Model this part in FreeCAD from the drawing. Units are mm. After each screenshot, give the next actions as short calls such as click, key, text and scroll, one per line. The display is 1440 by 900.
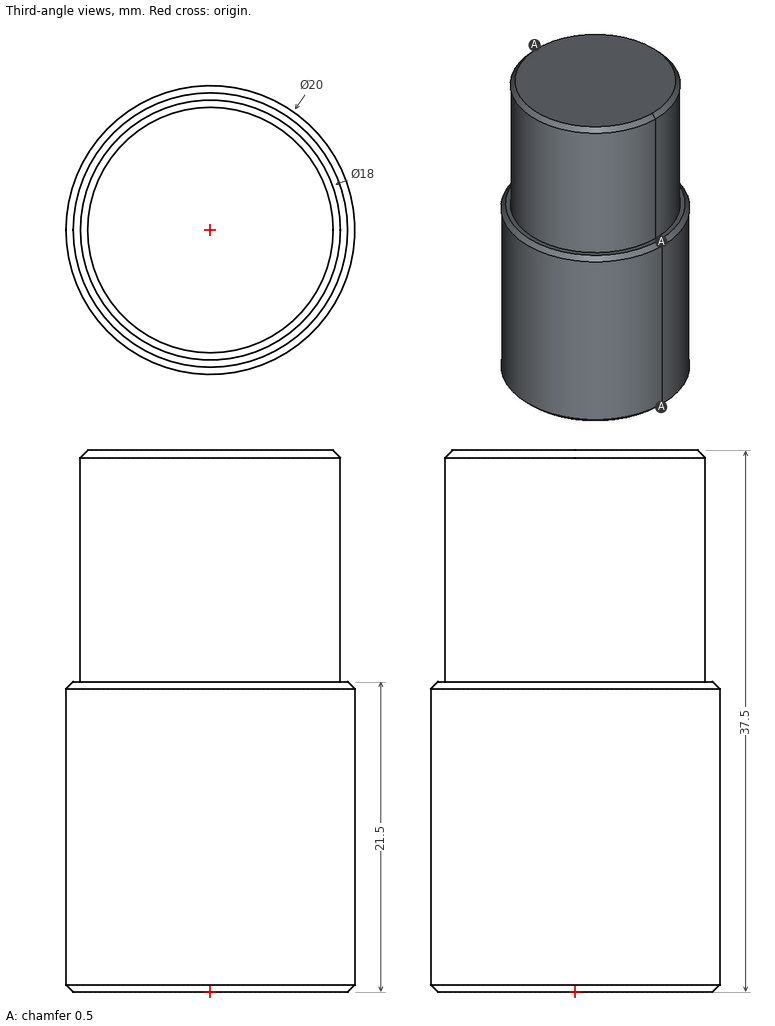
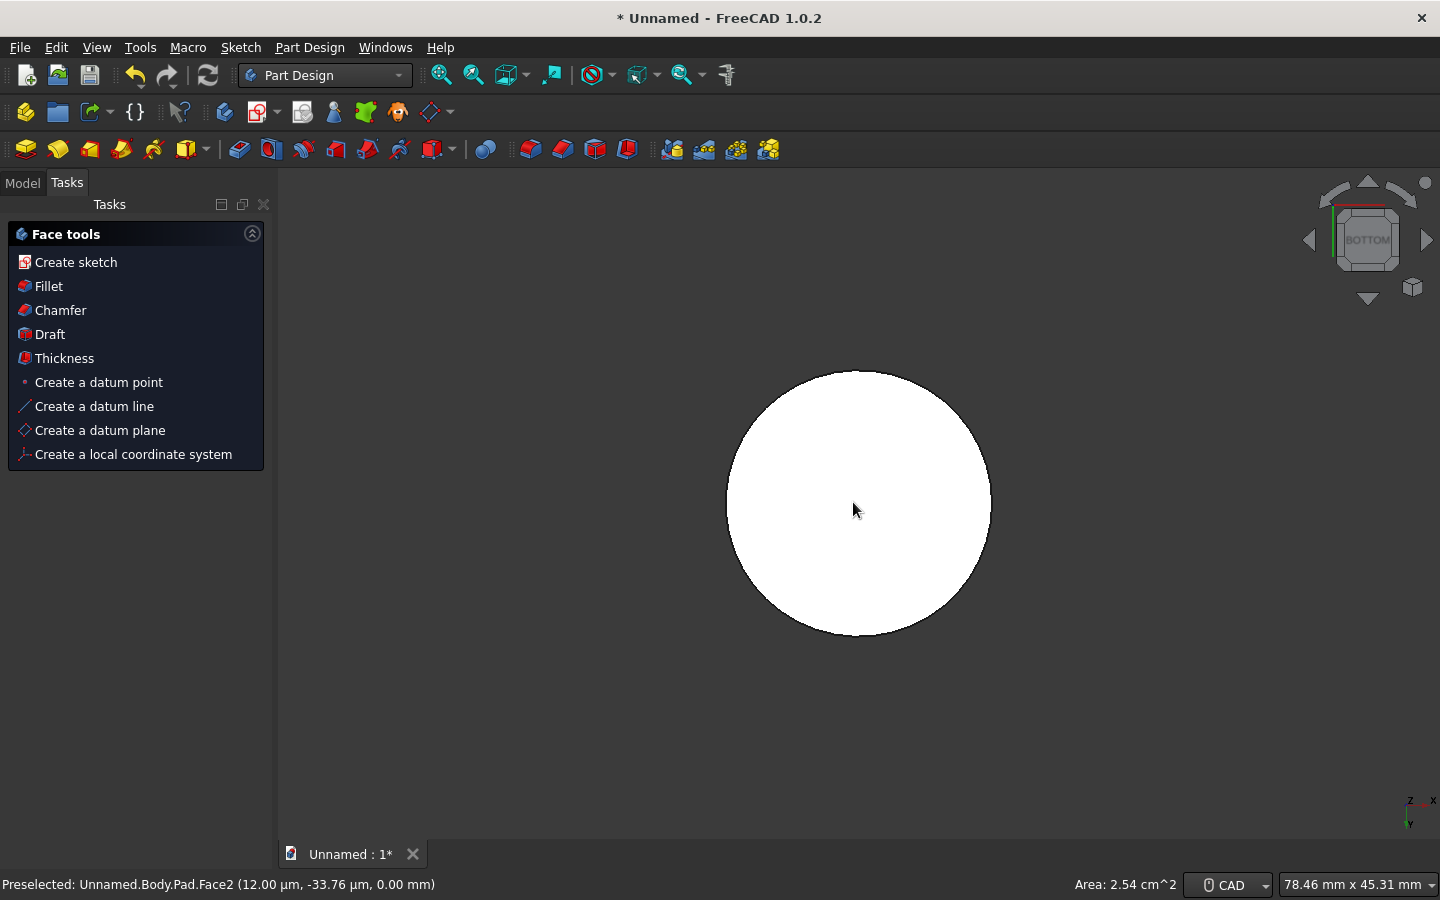
click(258, 112)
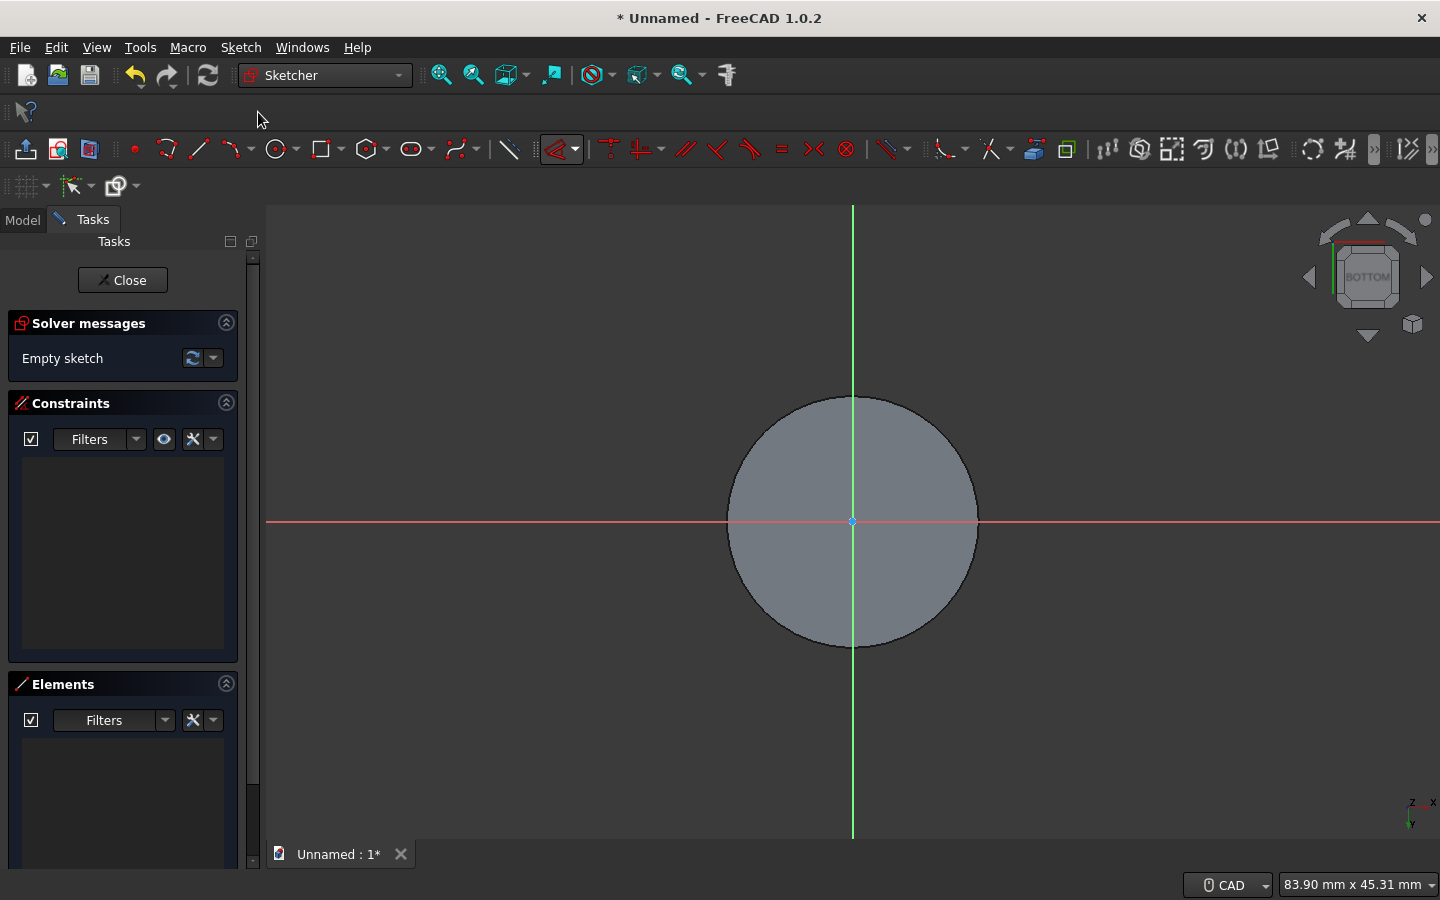
scroll(992, 522, up, 2)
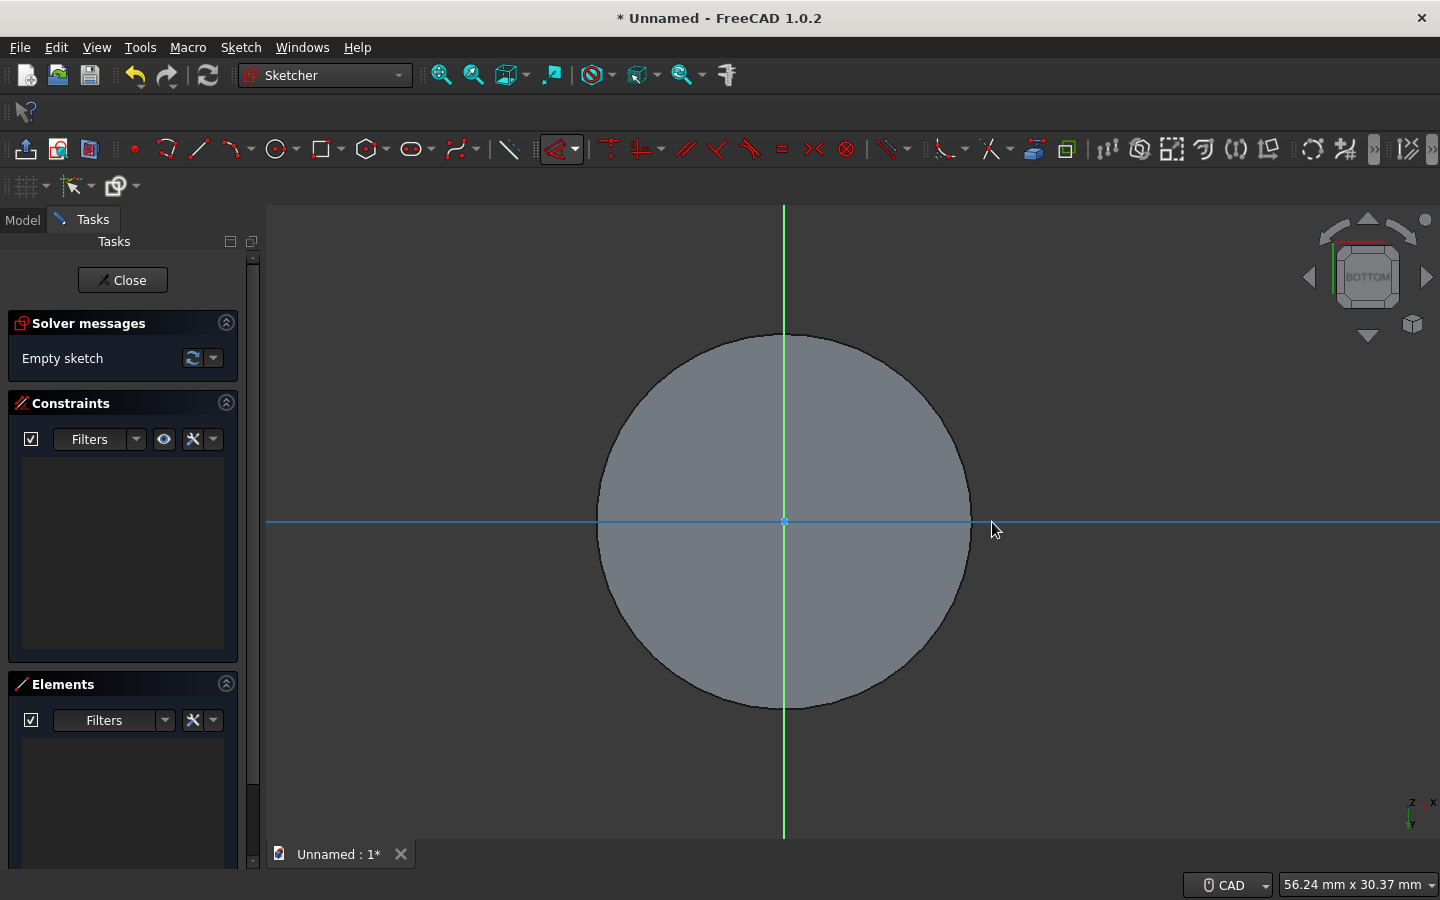
click(276, 150)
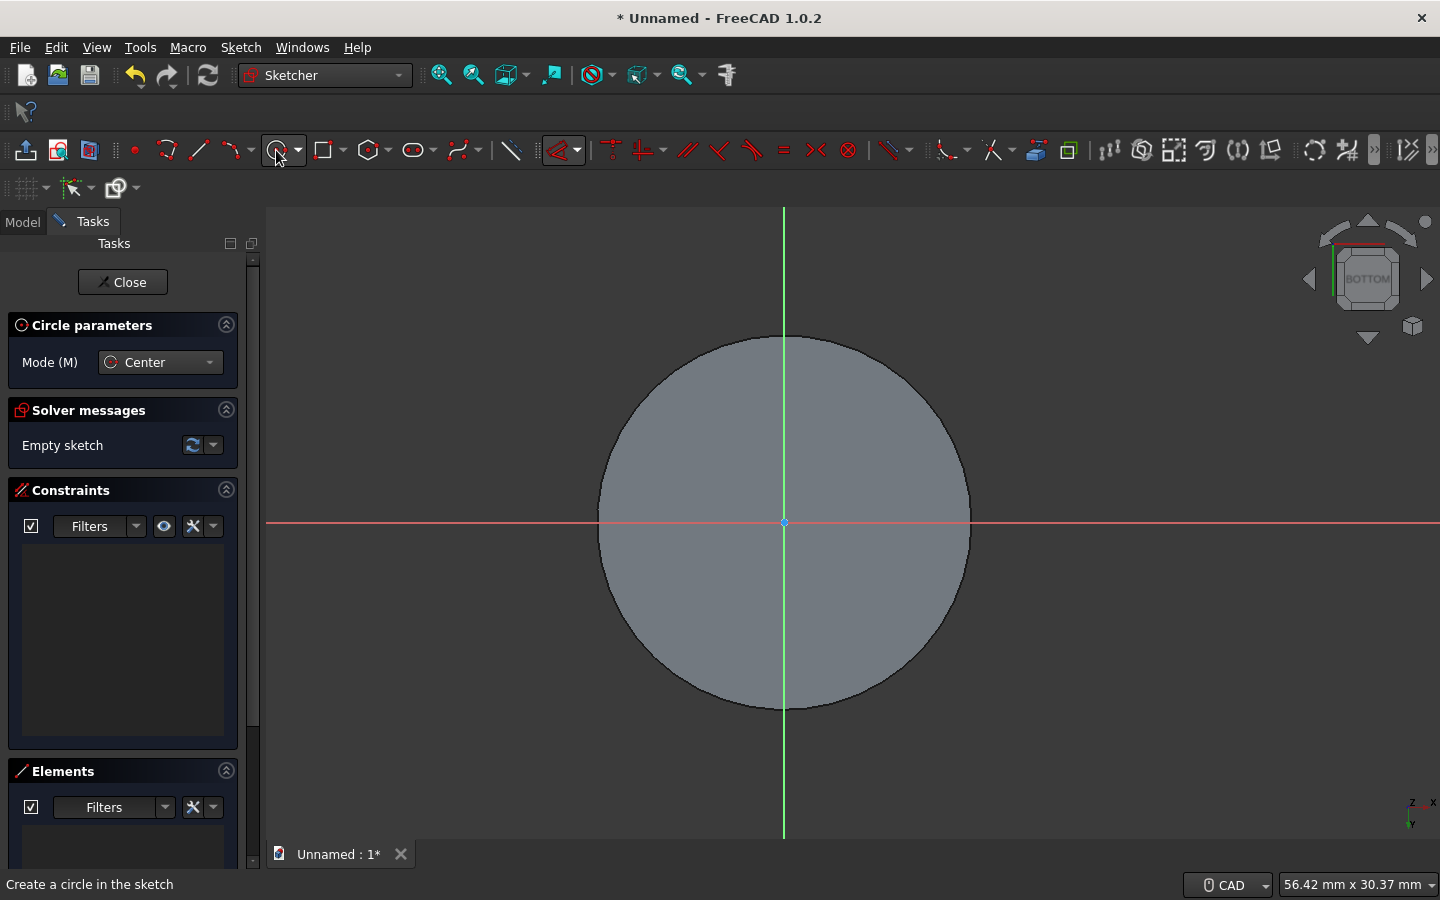
click(784, 523)
move(931, 376)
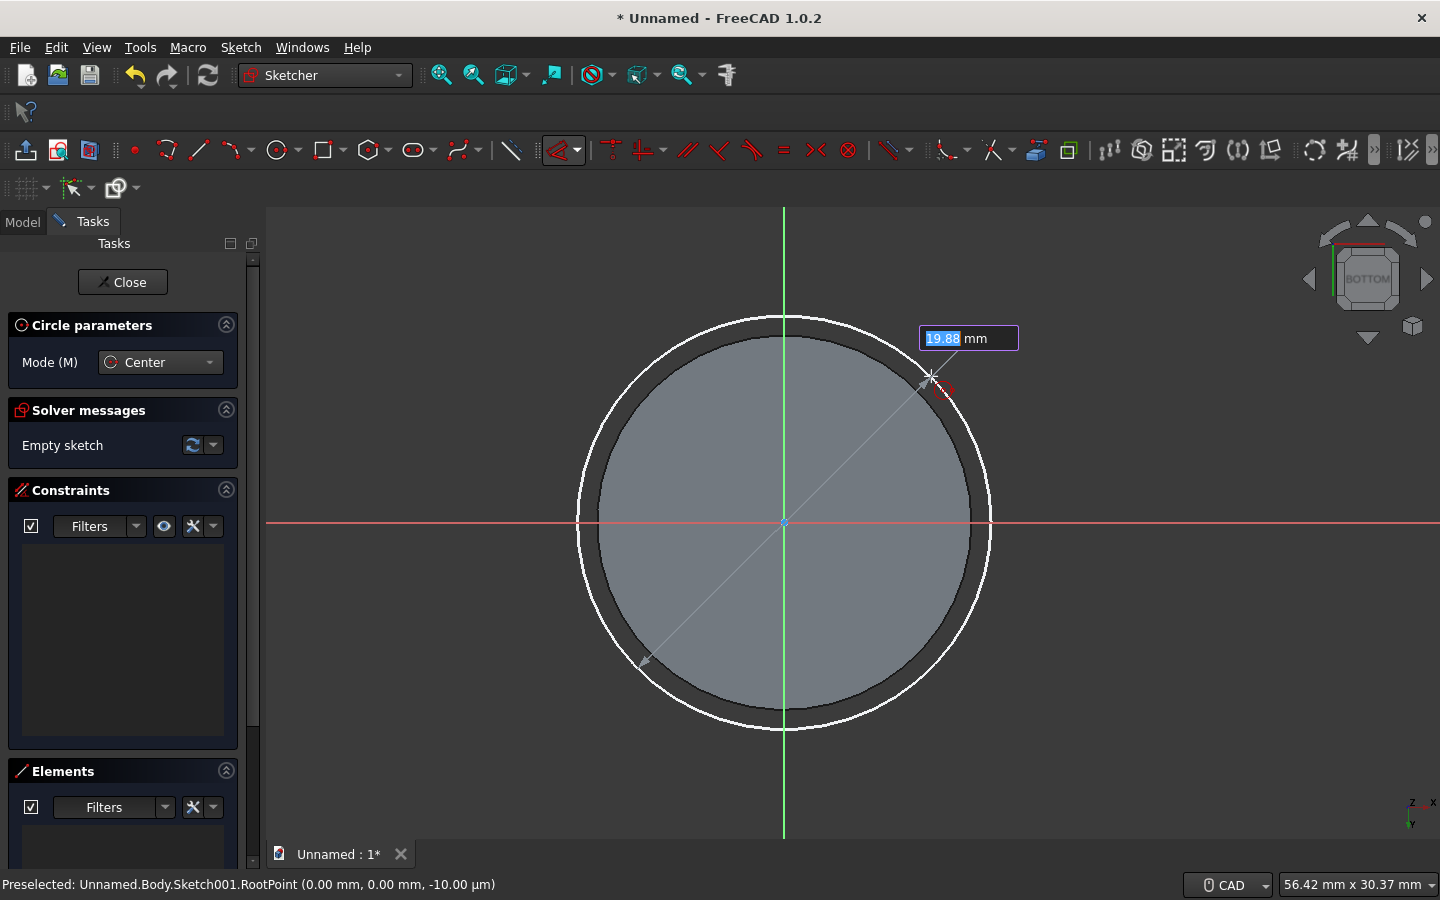
text(20)
key(Return)
key(Escape)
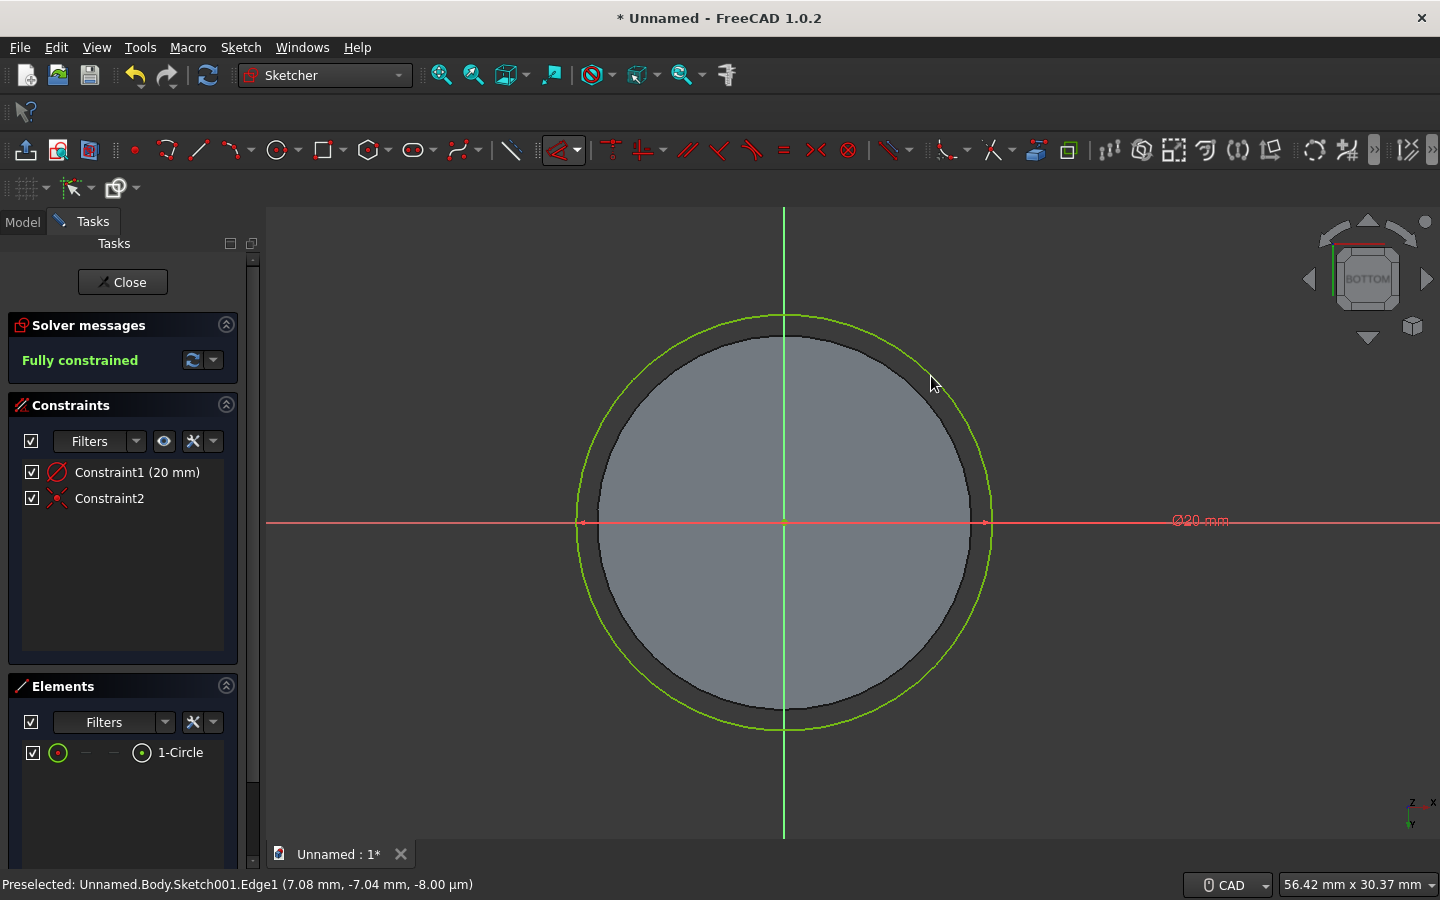
click(123, 282)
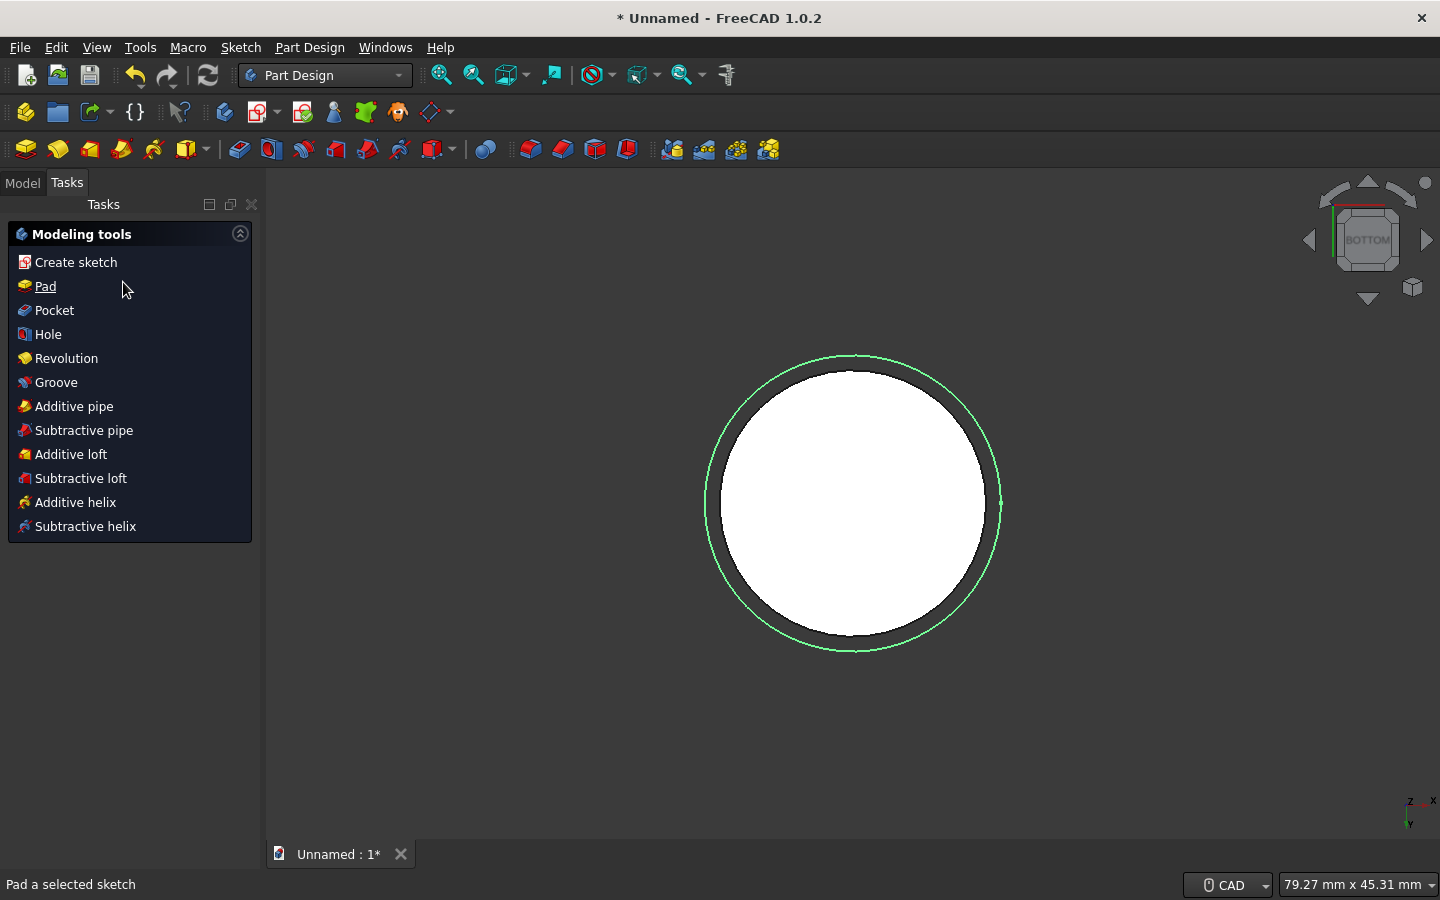
click(26, 150)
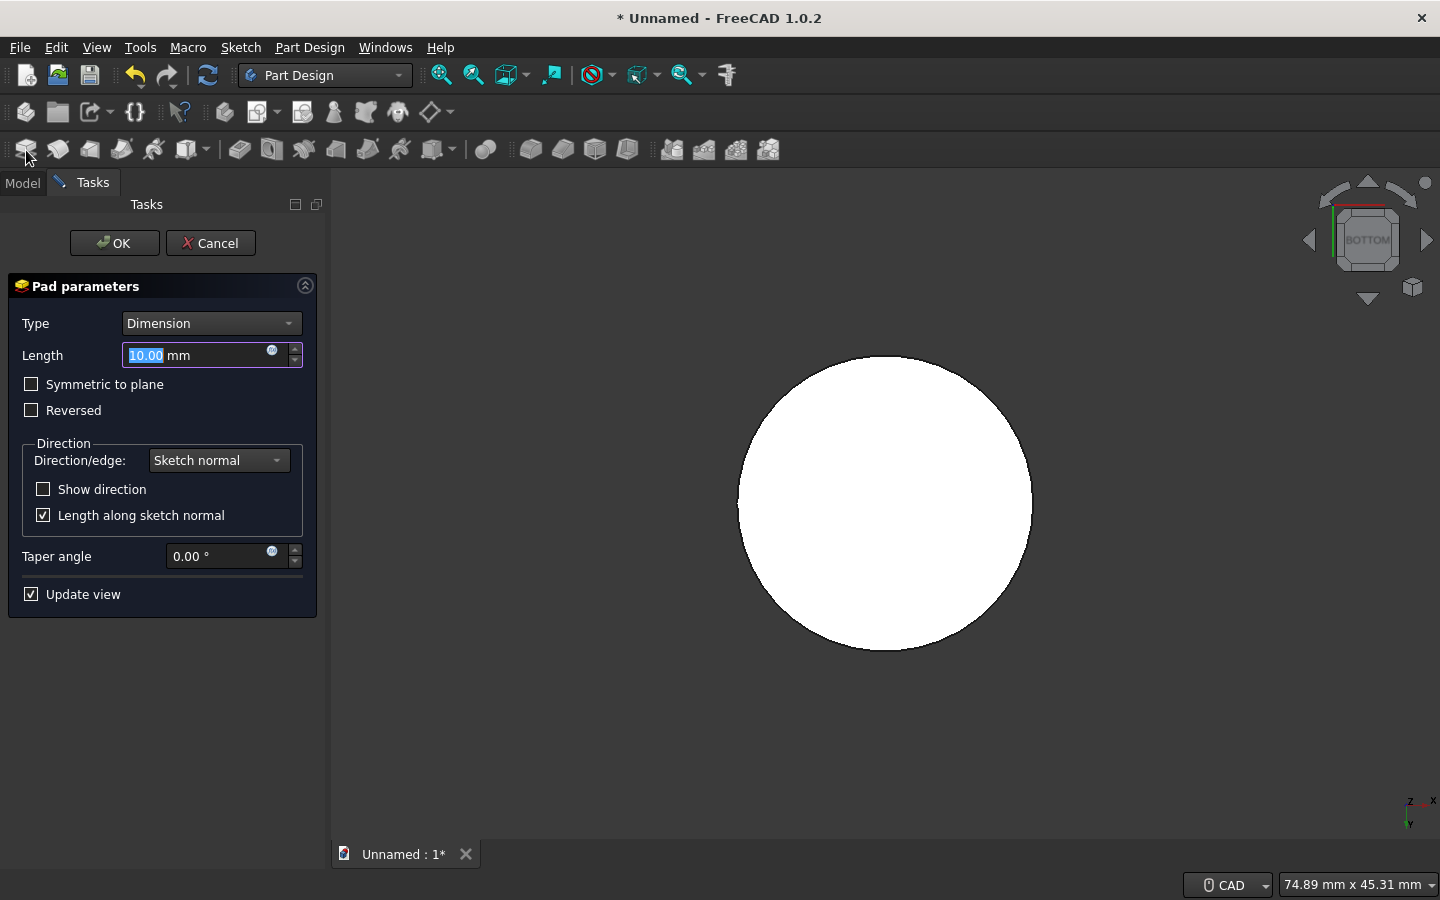
text(21.5)
key(Tab)